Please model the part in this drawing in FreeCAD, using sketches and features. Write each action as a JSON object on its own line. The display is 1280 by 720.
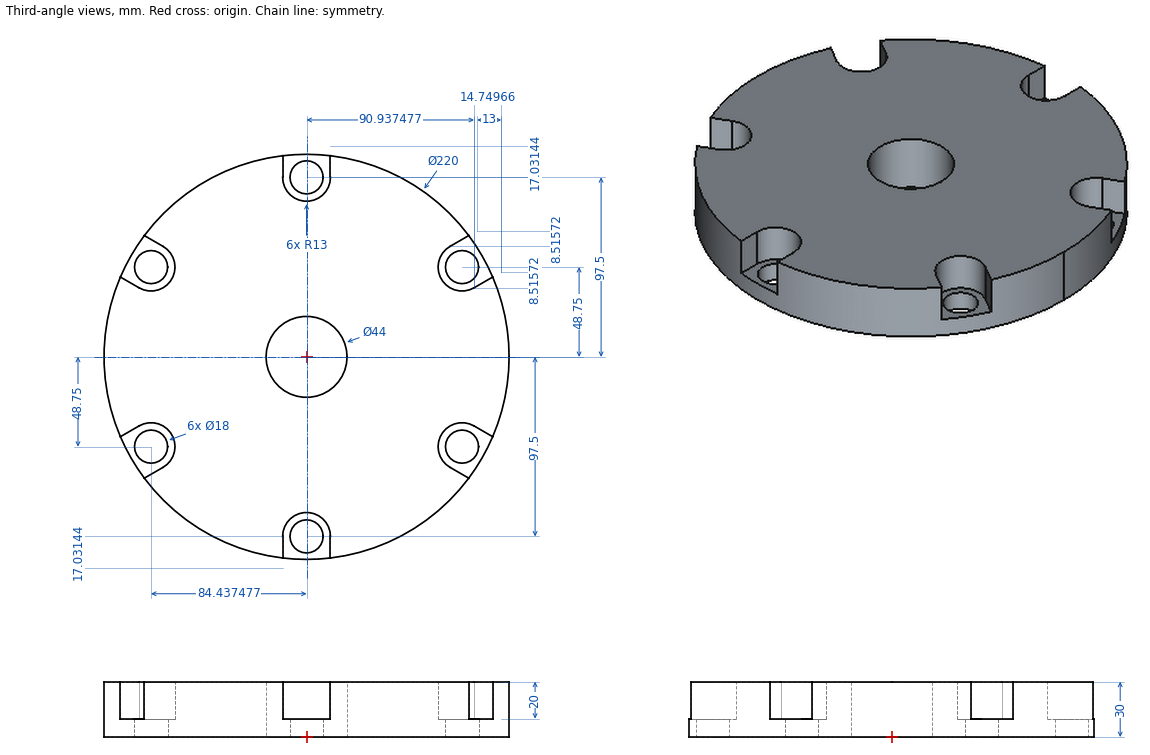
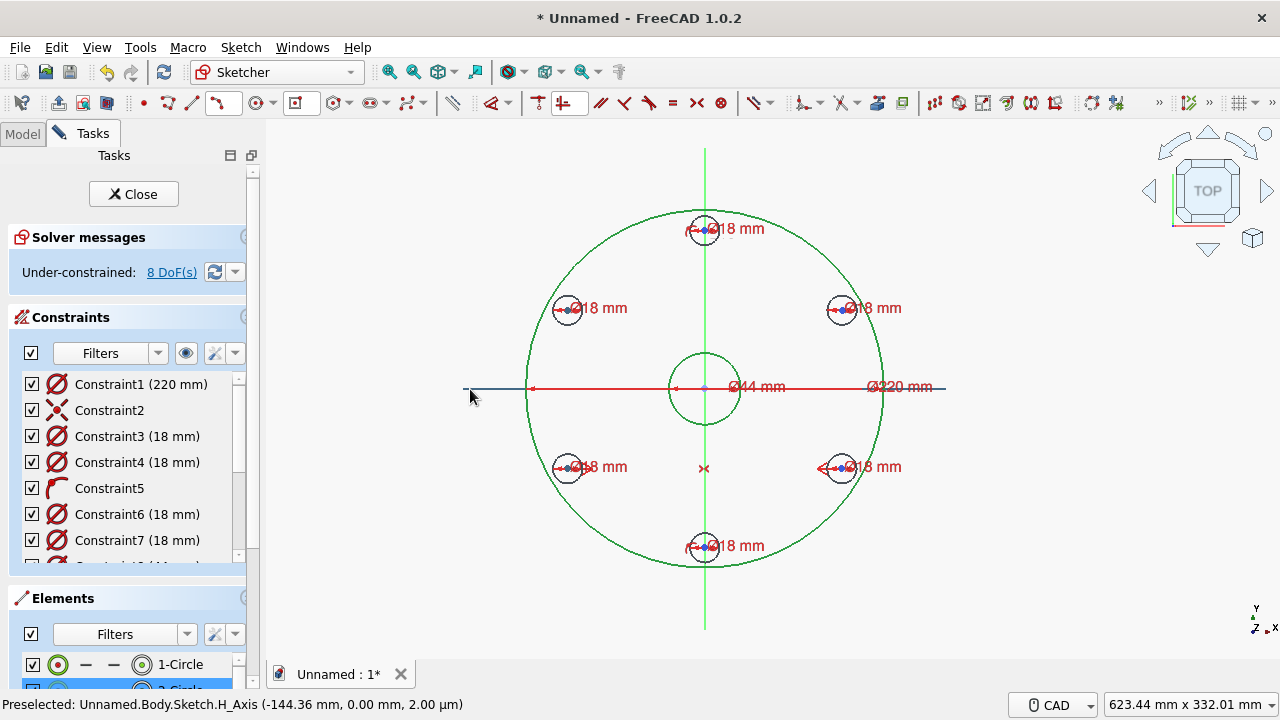
{"action": "left_click", "coordinate": [698, 104]}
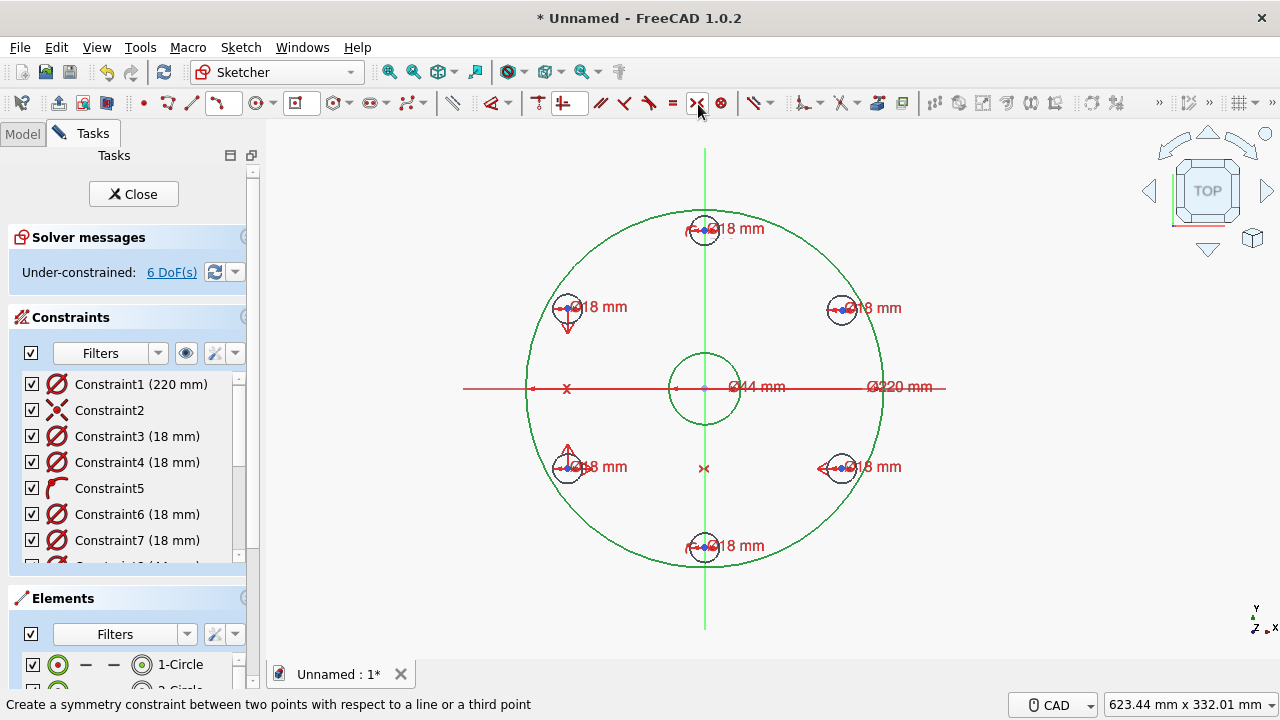
{"action": "left_click", "coordinate": [842, 469]}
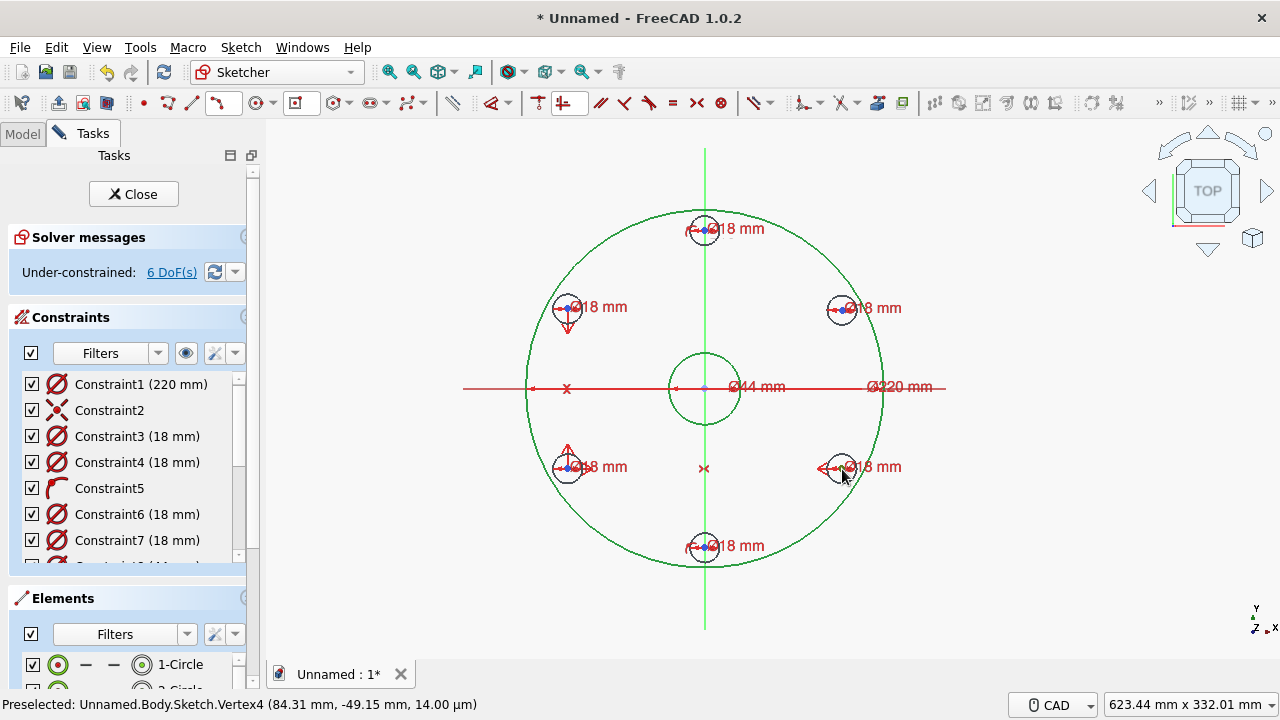
{"action": "left_click", "coordinate": [842, 310]}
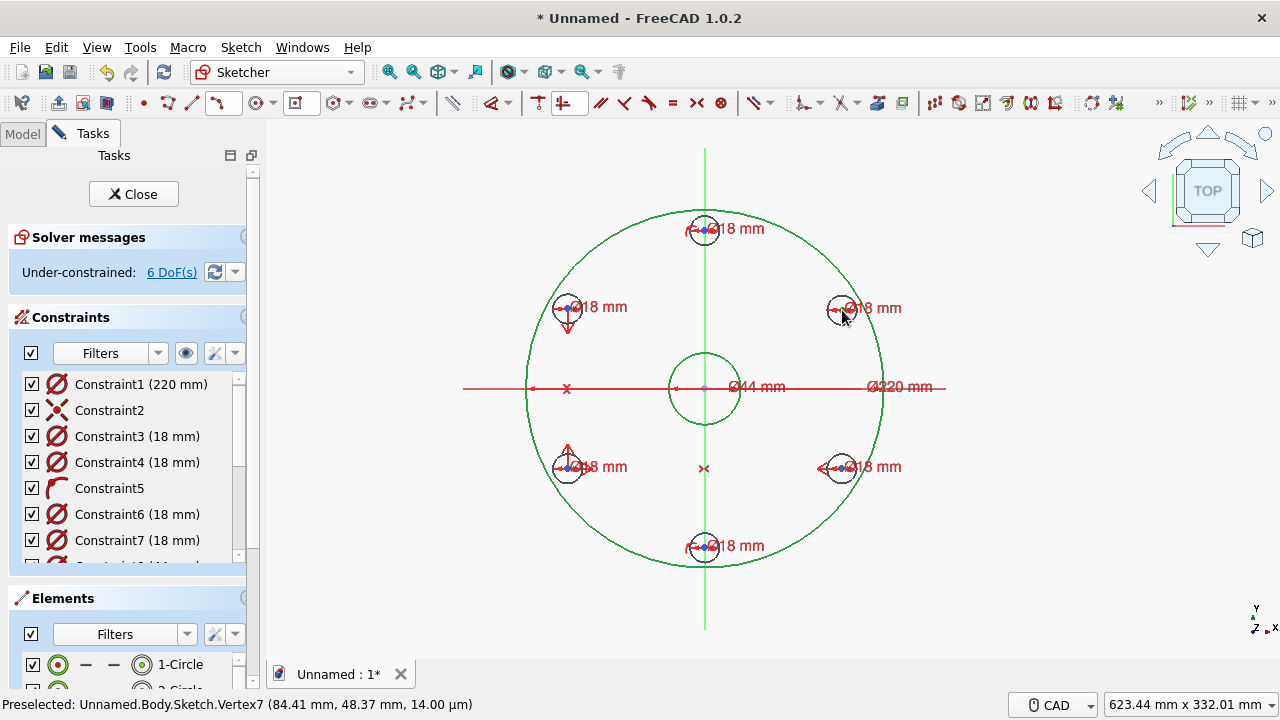
{"action": "left_click", "coordinate": [470, 389]}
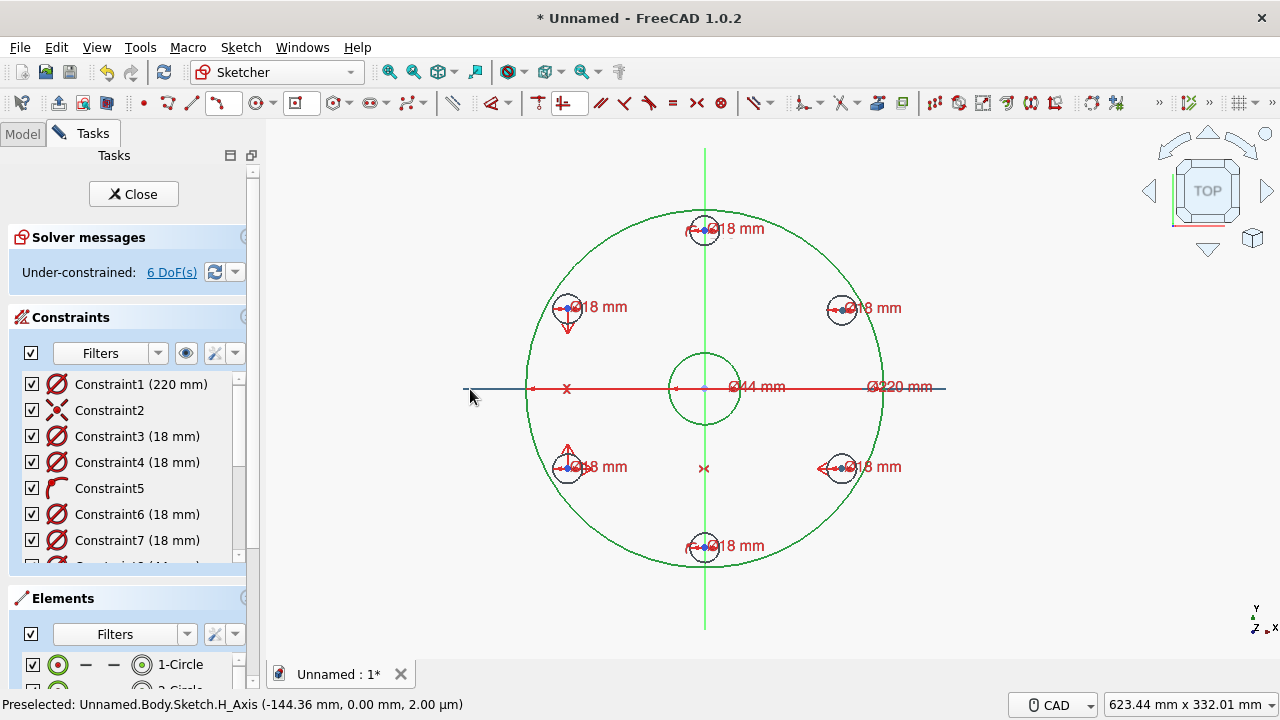
{"action": "left_click", "coordinate": [698, 104]}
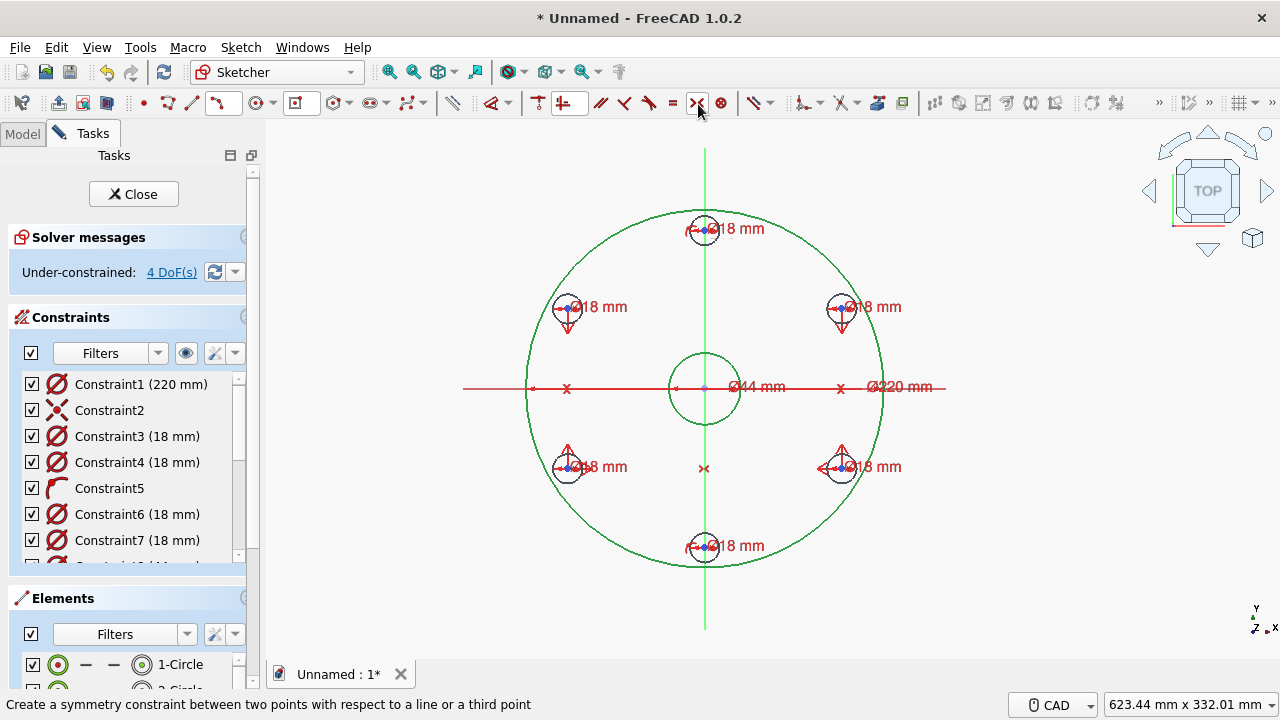
{"action": "left_click", "coordinate": [705, 548]}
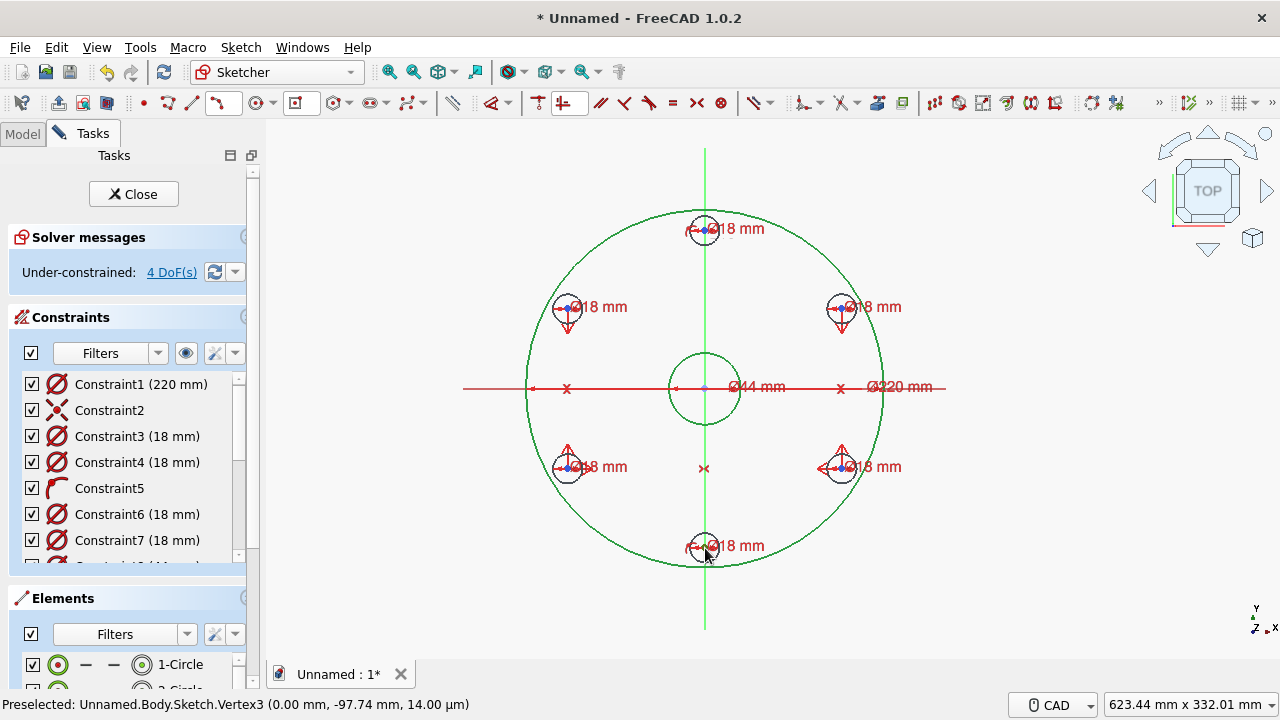
{"action": "key", "text": "i"}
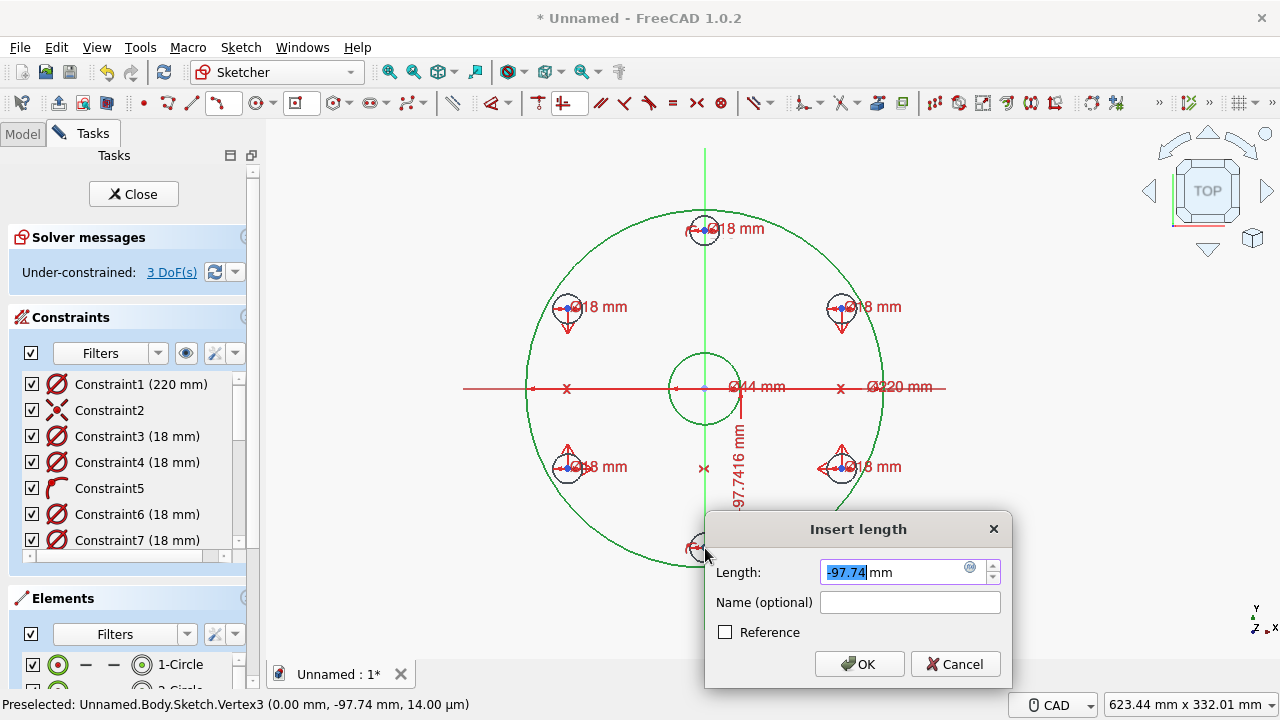
{"action": "type", "text": "-97.5"}
{"action": "key", "text": "Return"}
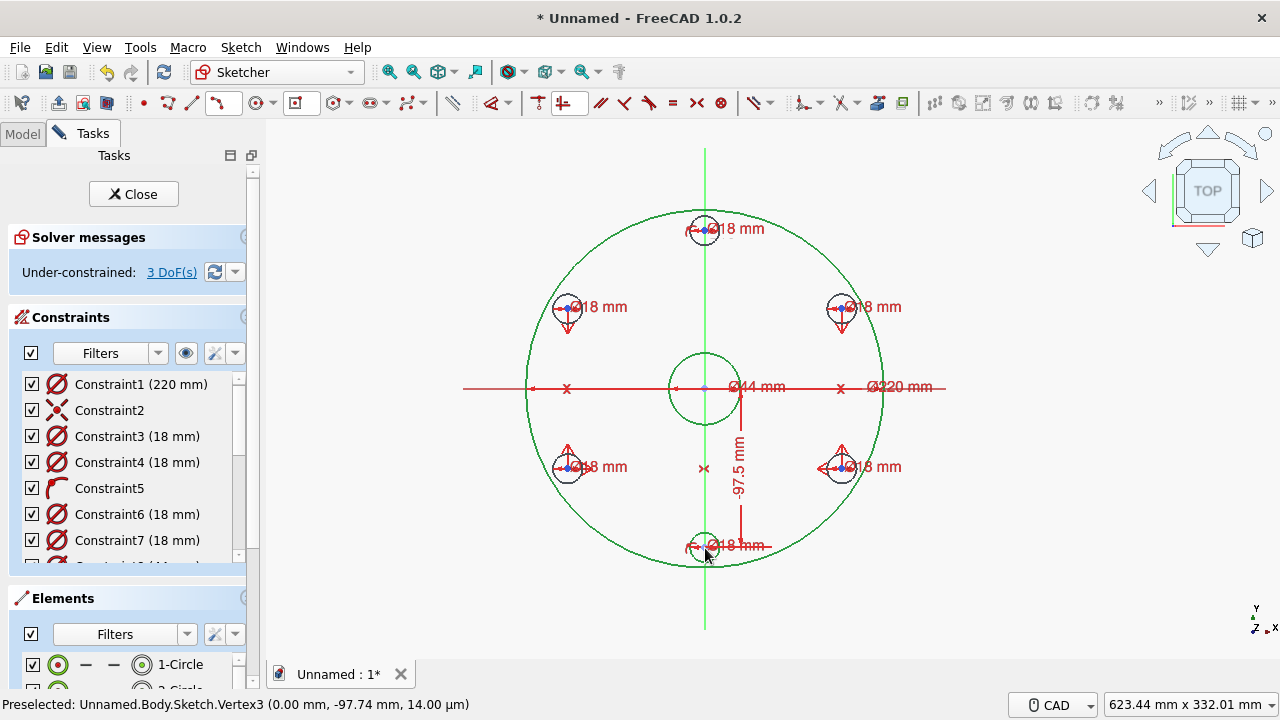
{"action": "left_click", "coordinate": [705, 231]}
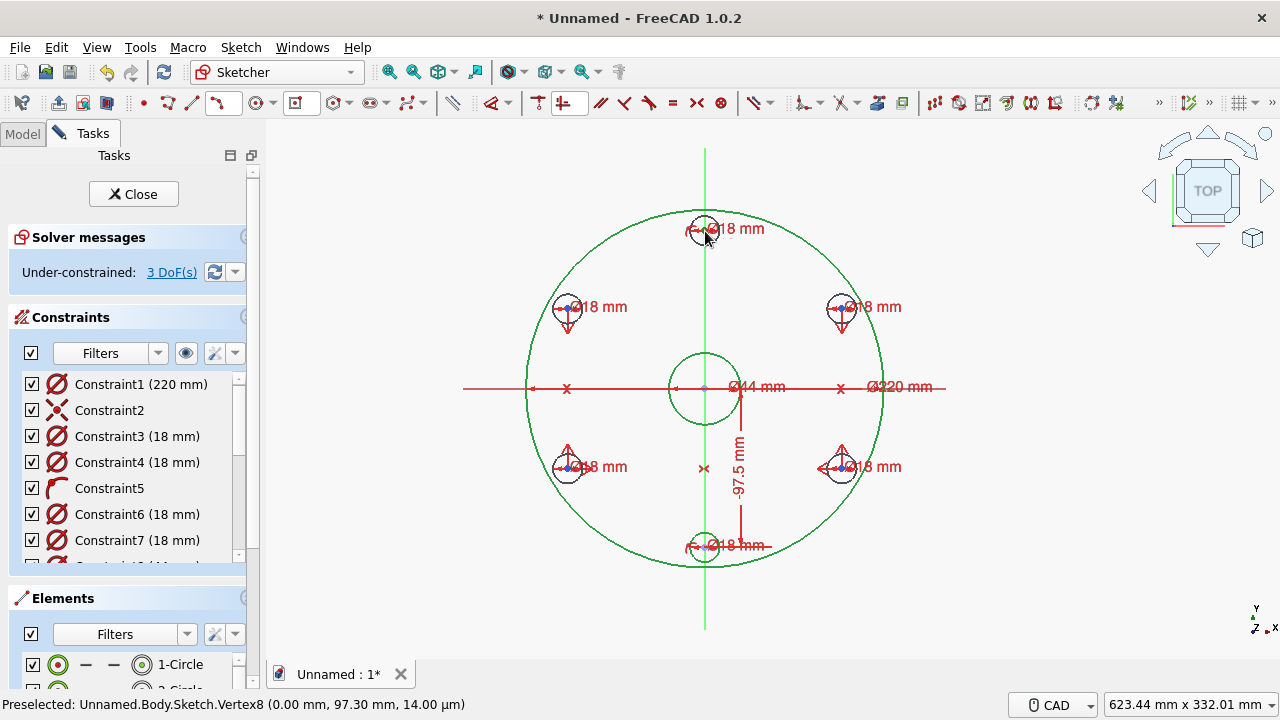
{"action": "key", "text": "i"}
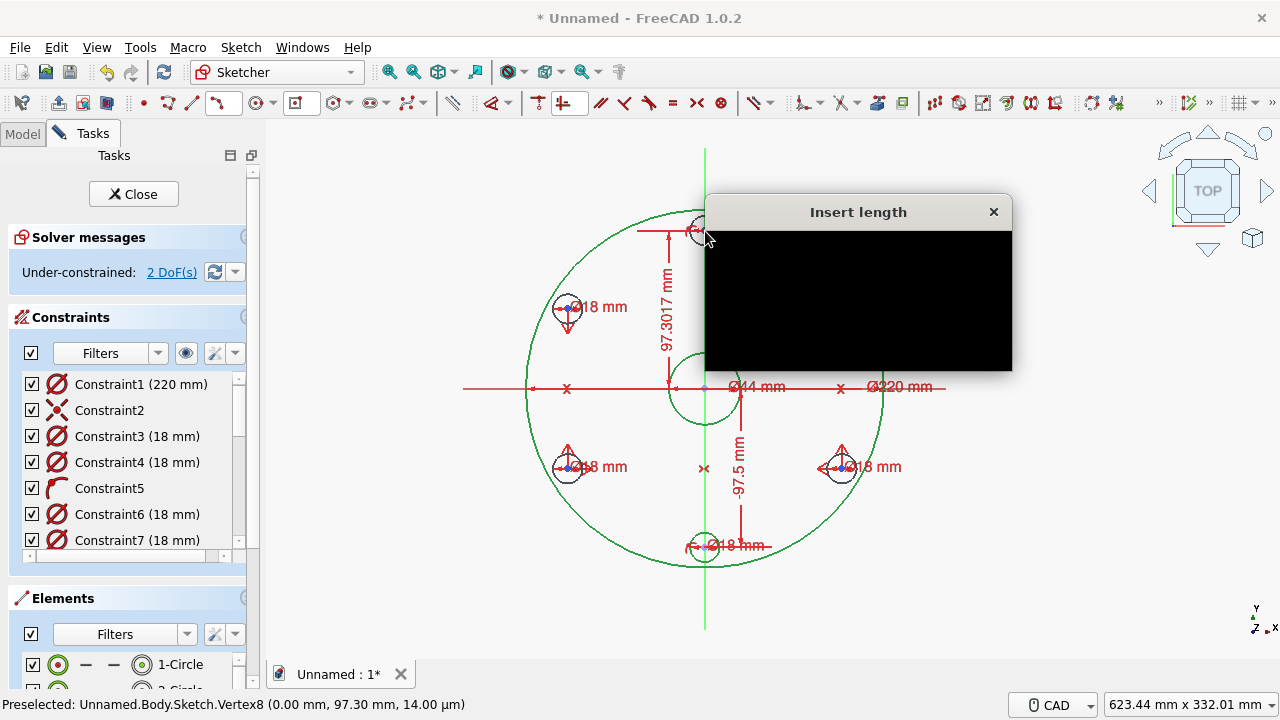
{"action": "type", "text": "97.5"}
{"action": "key", "text": "Return"}